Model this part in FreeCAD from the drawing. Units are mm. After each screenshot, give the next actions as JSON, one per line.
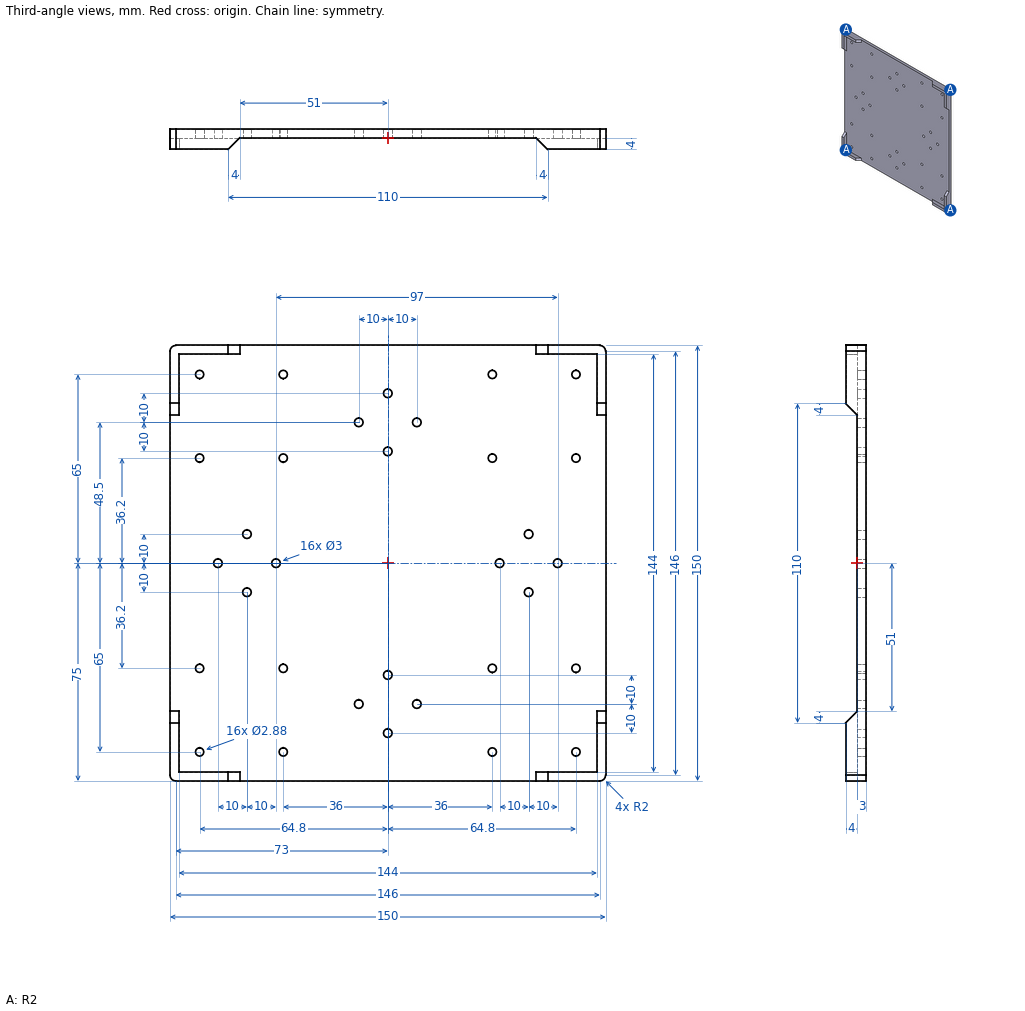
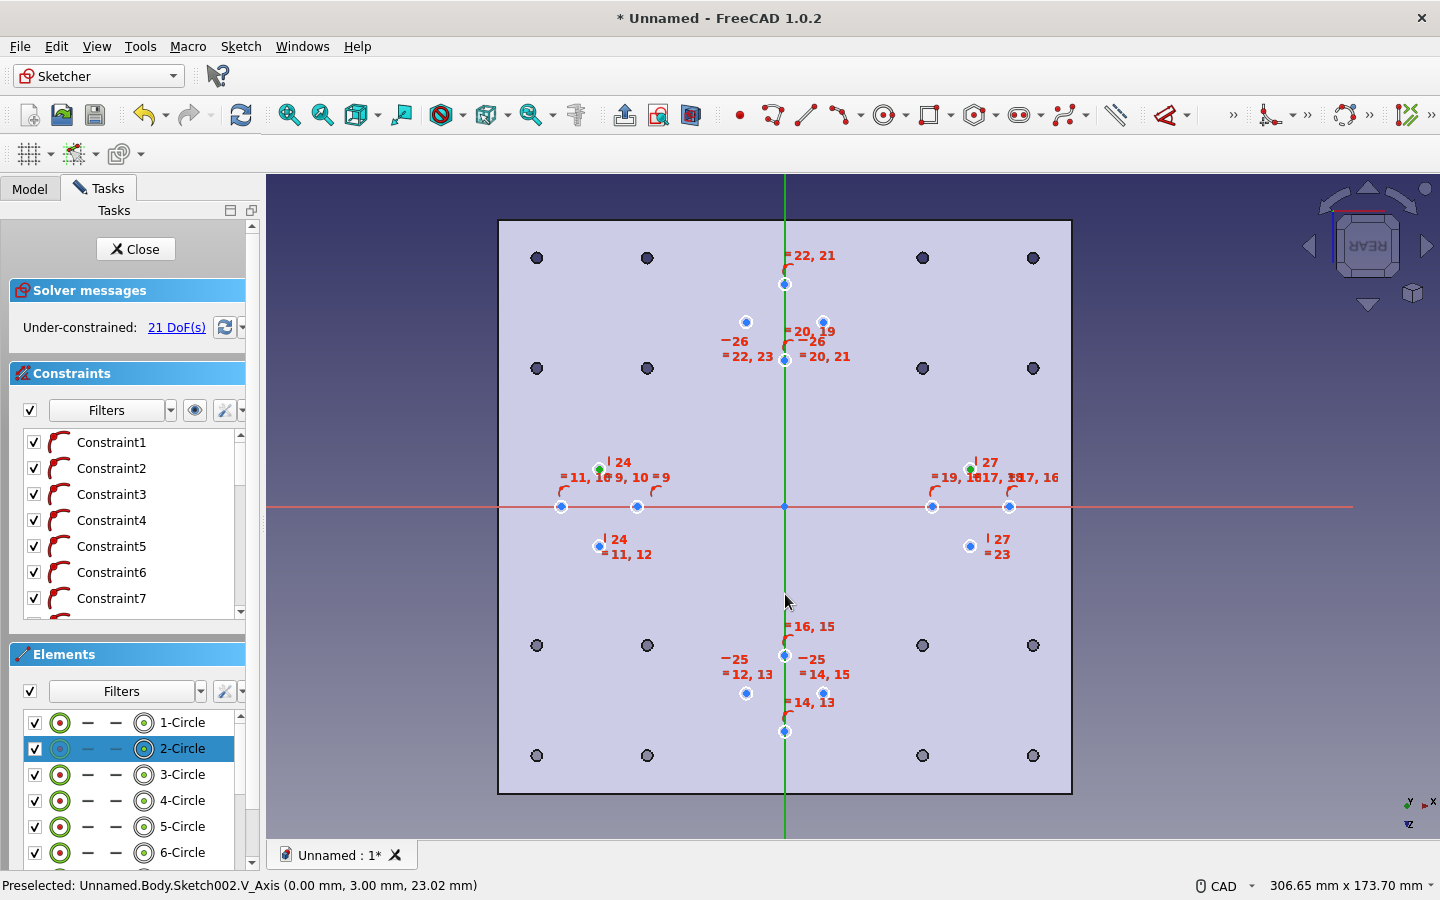
{"action": "key", "text": "s"}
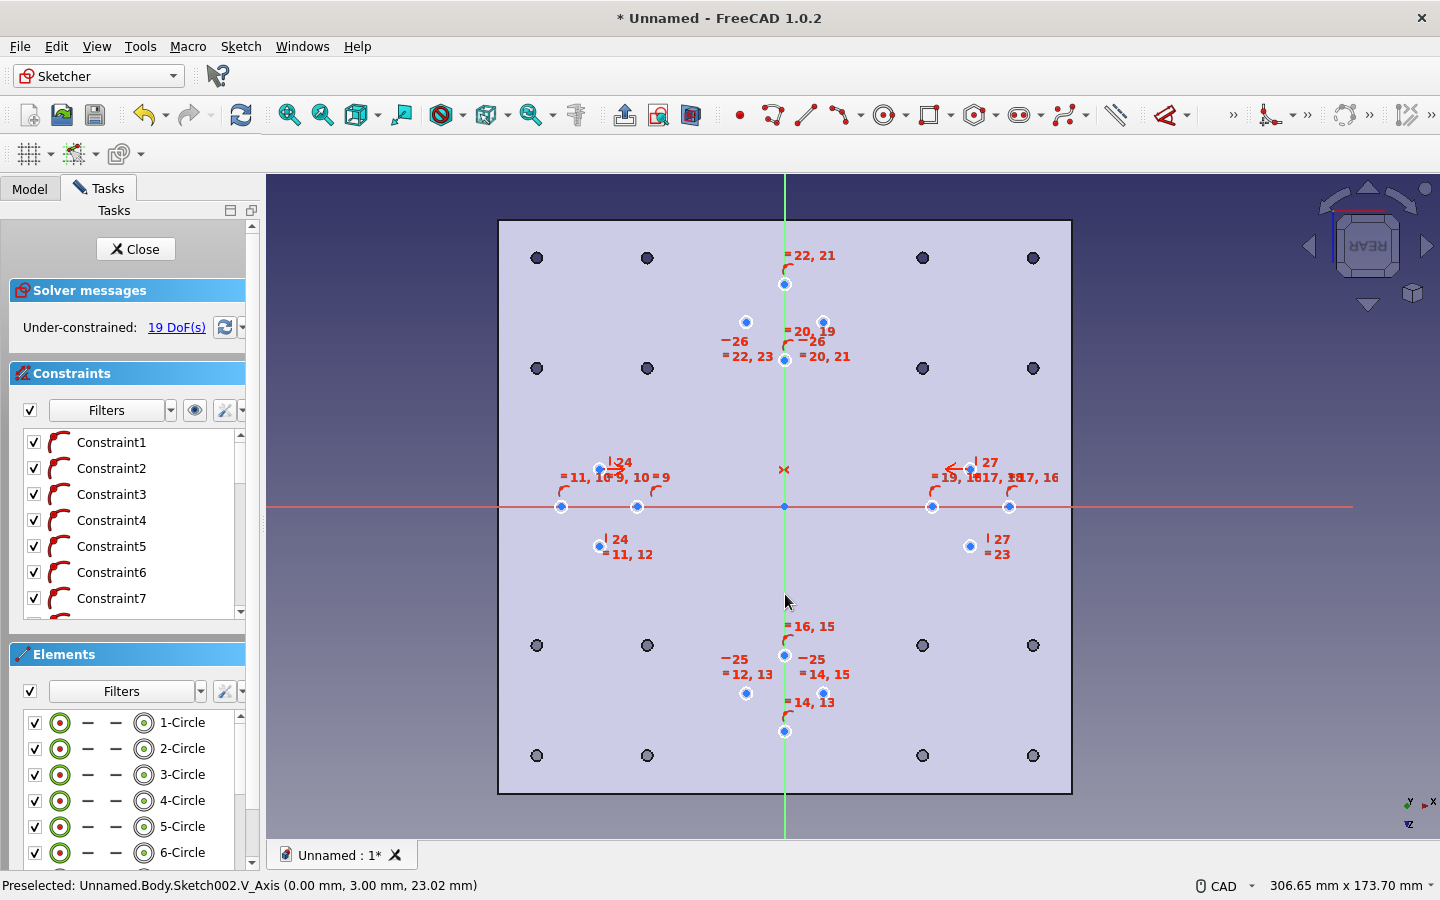
{"action": "left_click", "coordinate": [823, 694]}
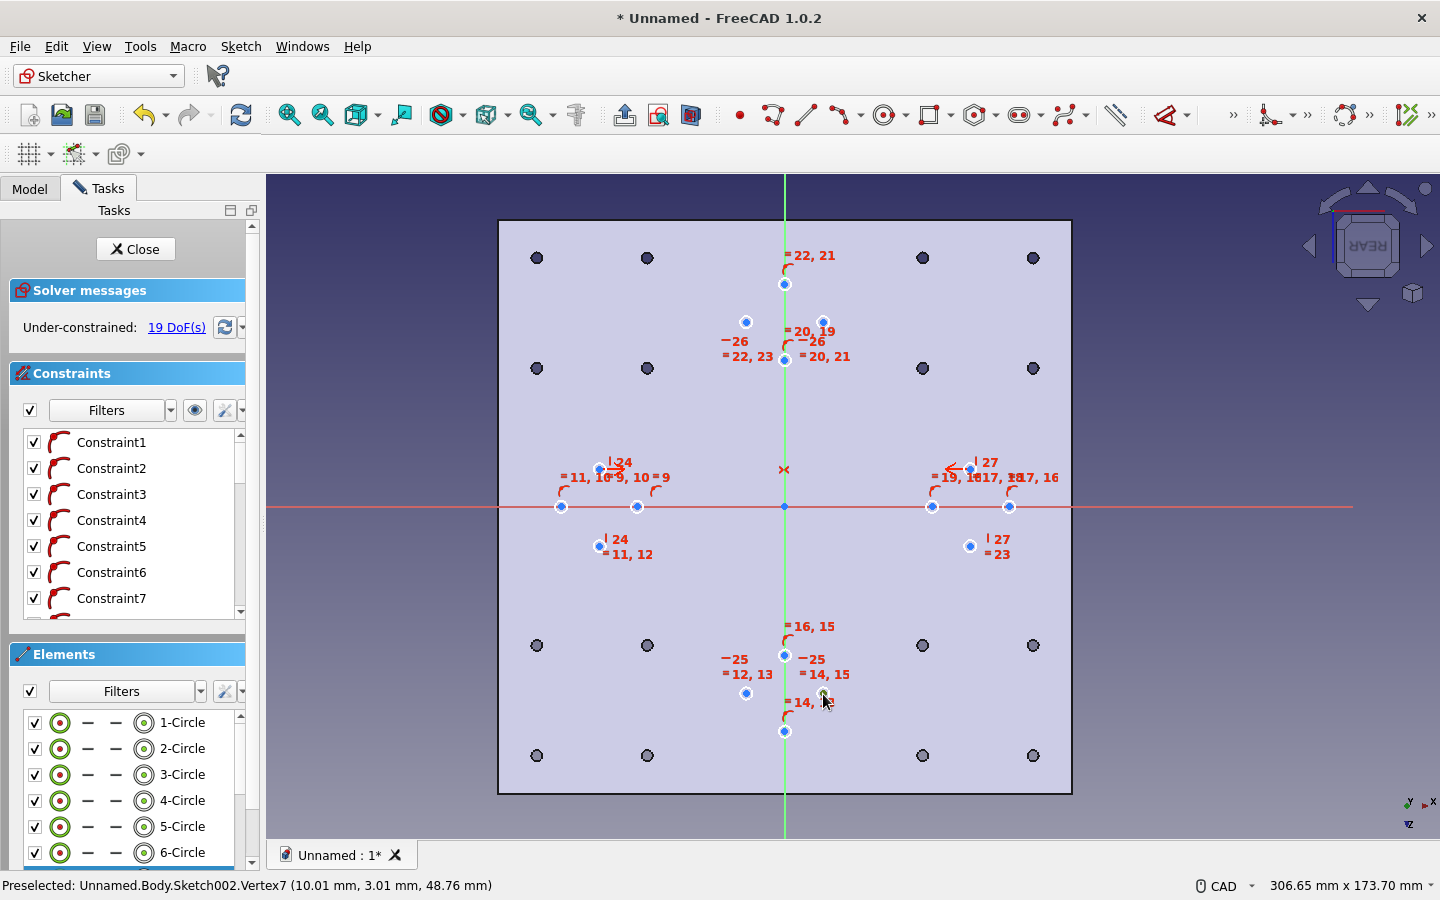
{"action": "left_click", "coordinate": [823, 322]}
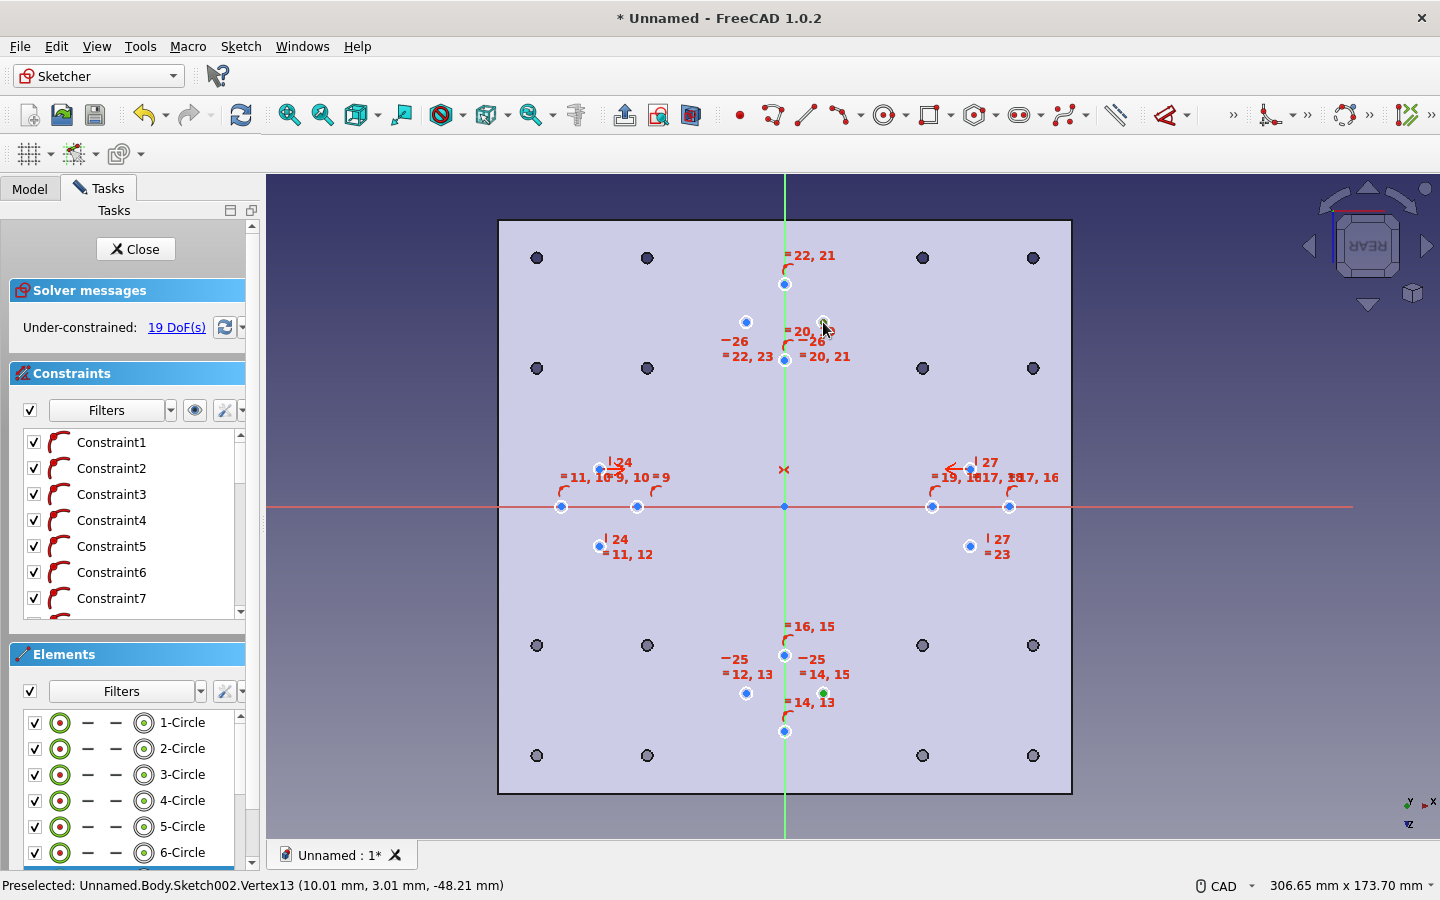
{"action": "left_click", "coordinate": [364, 507]}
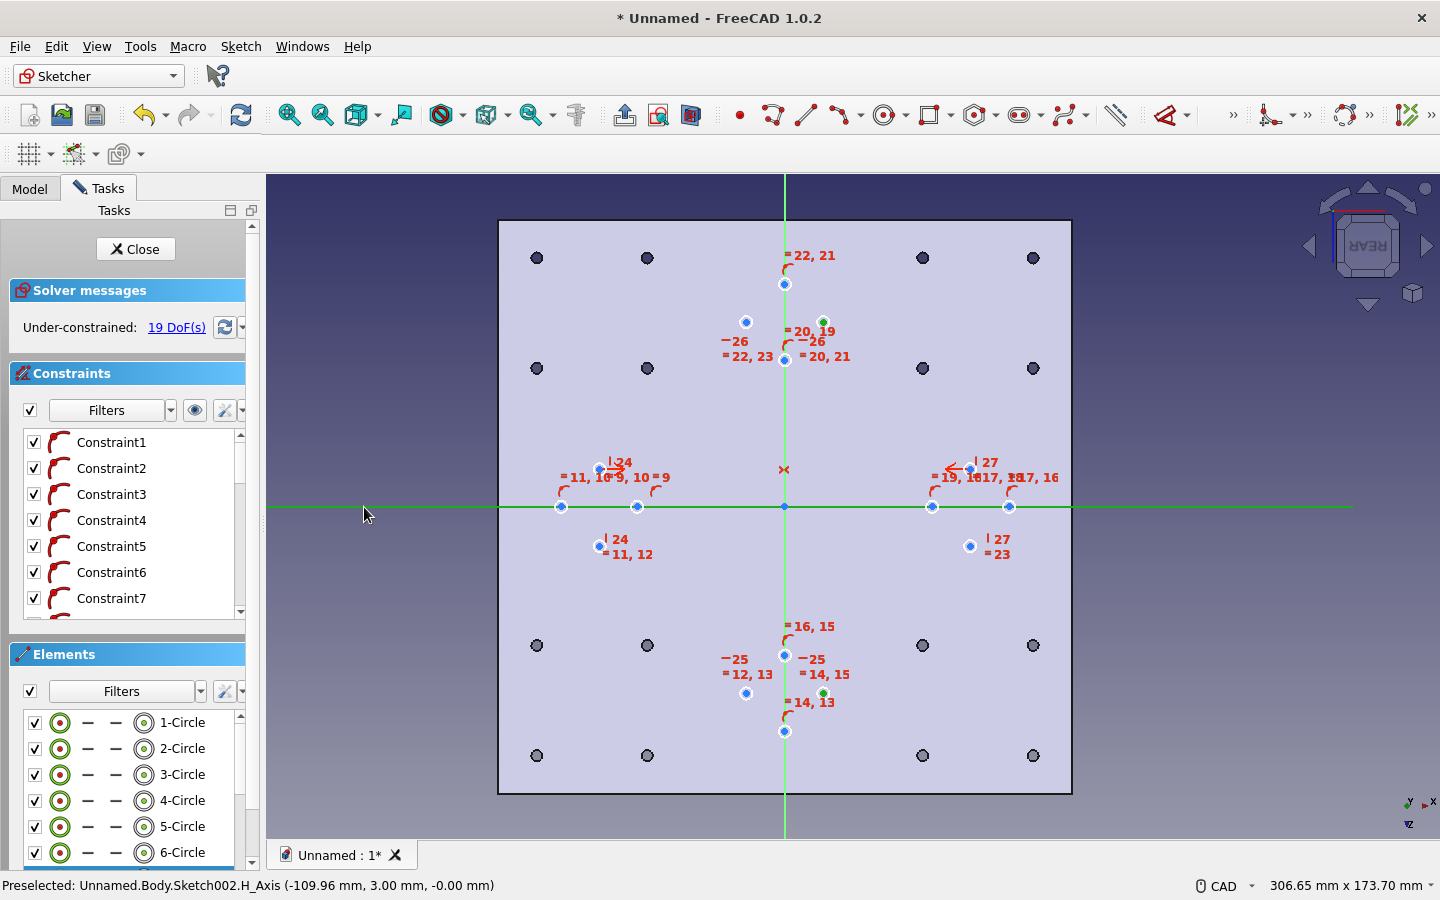
{"action": "key", "text": "s"}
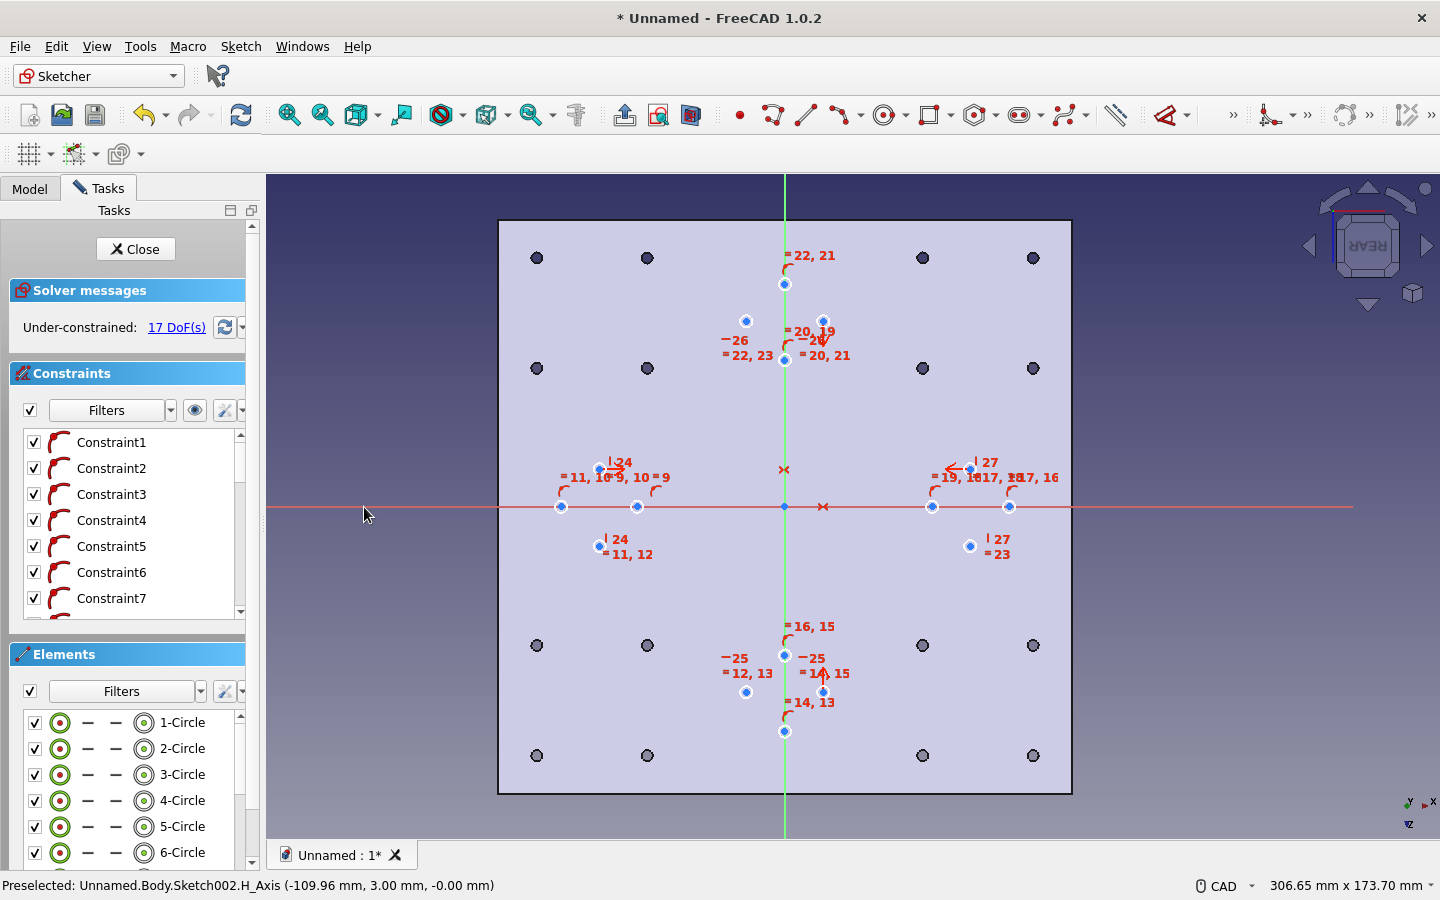
{"action": "left_click", "coordinate": [1164, 116]}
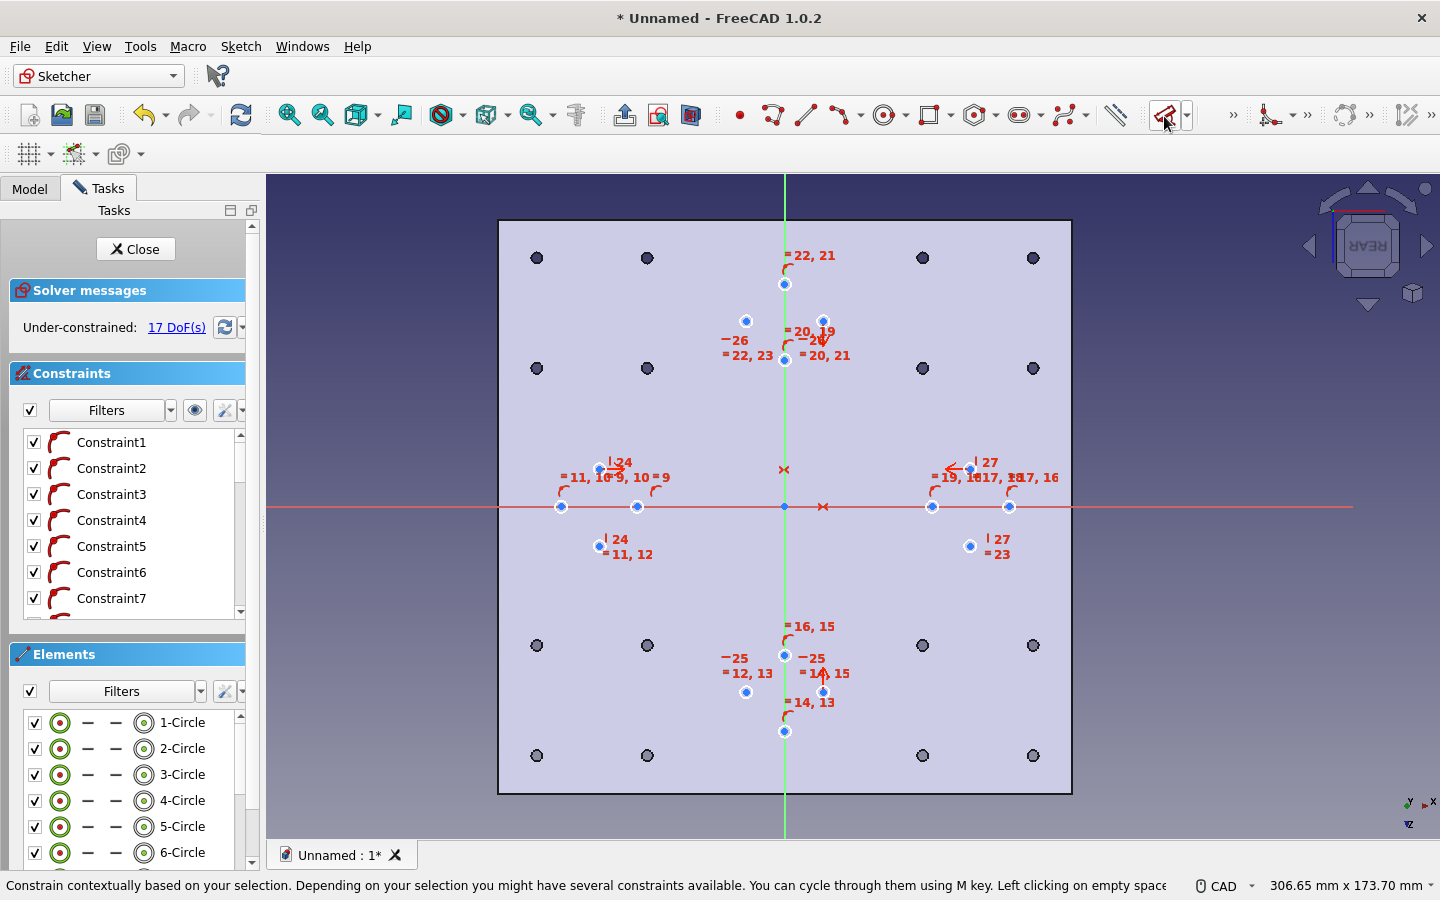
{"action": "scroll", "coordinate": [643, 507], "scroll_direction": "up", "scroll_amount": 7}